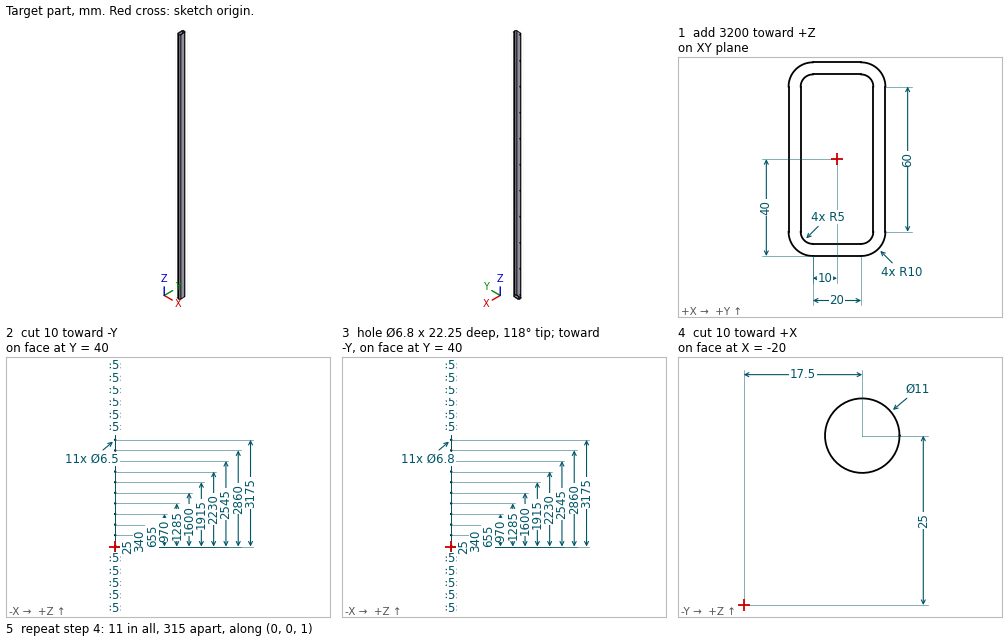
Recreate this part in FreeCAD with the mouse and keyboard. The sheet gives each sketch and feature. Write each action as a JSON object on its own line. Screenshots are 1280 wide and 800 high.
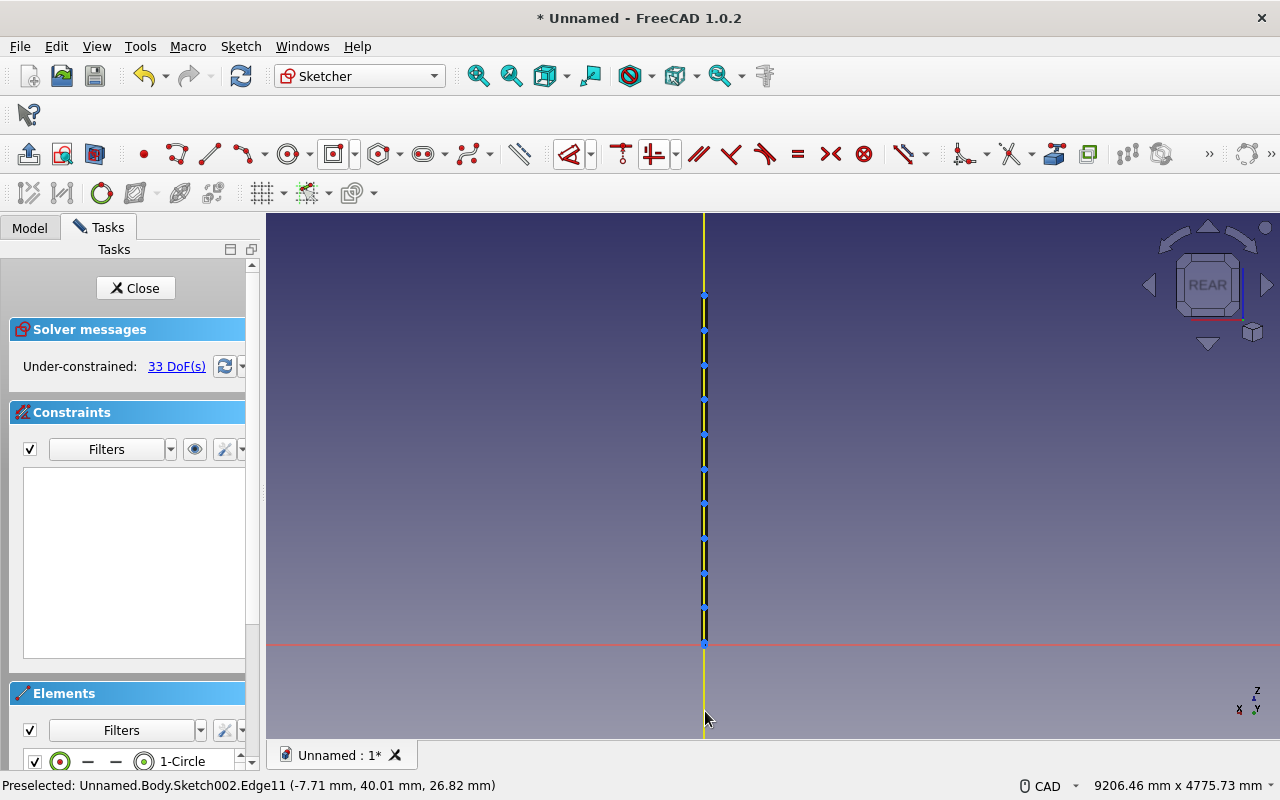
{"action": "scroll", "coordinate": [705, 295], "scroll_direction": "up", "scroll_amount": 14}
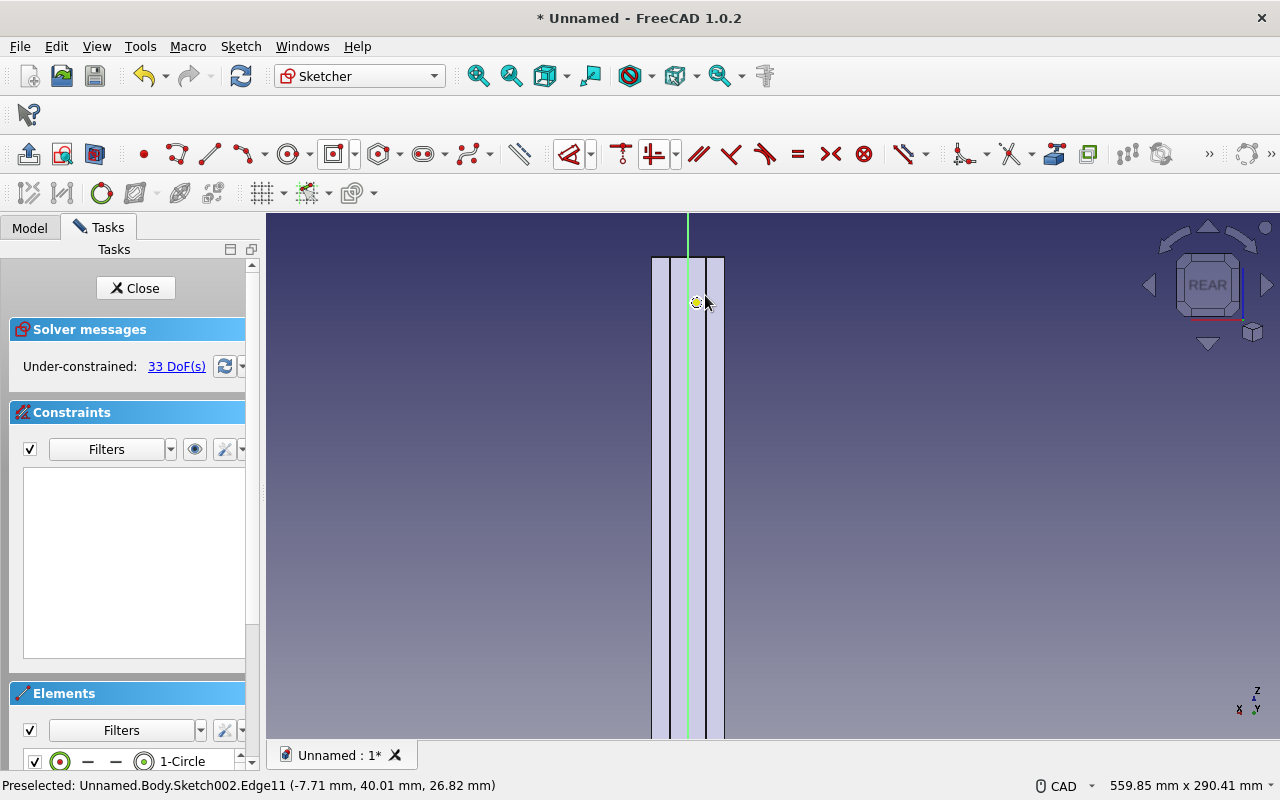
{"action": "left_click", "coordinate": [701, 298]}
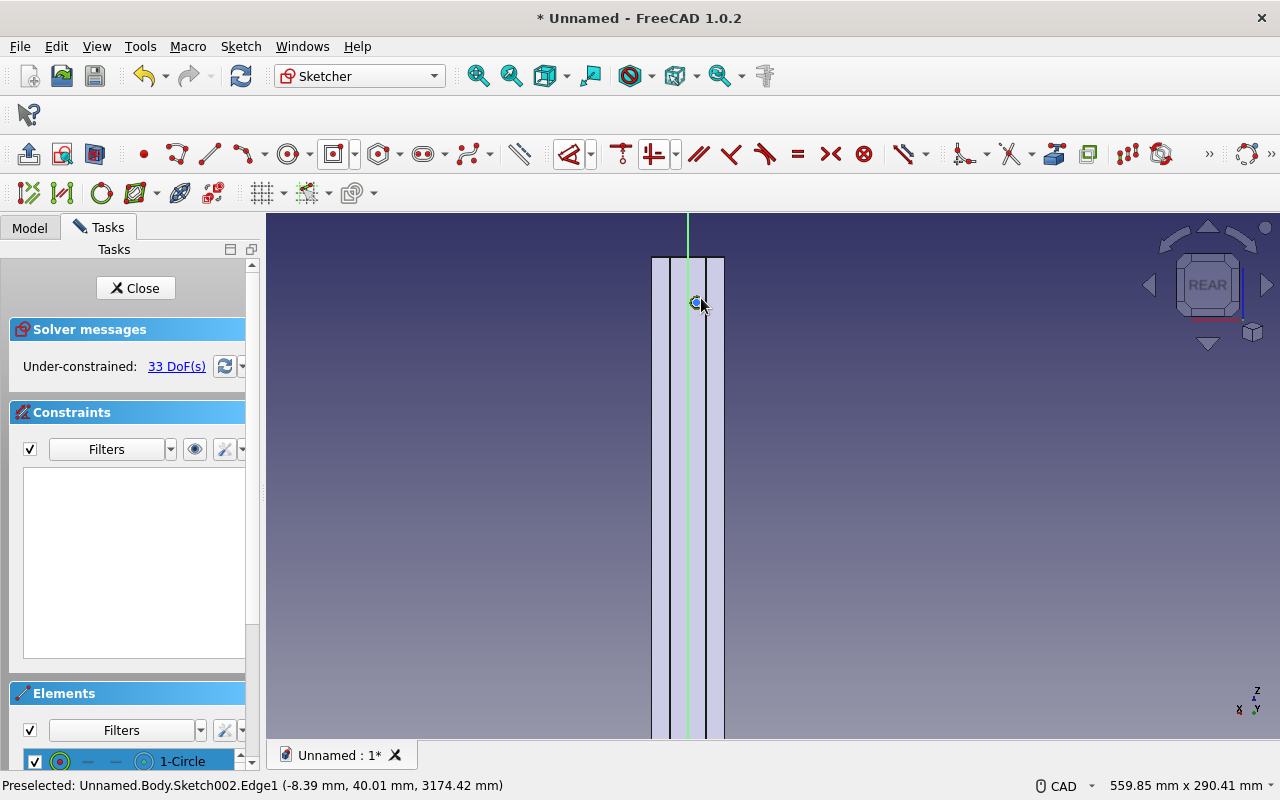
{"action": "scroll", "coordinate": [705, 301], "scroll_direction": "down", "scroll_amount": 14}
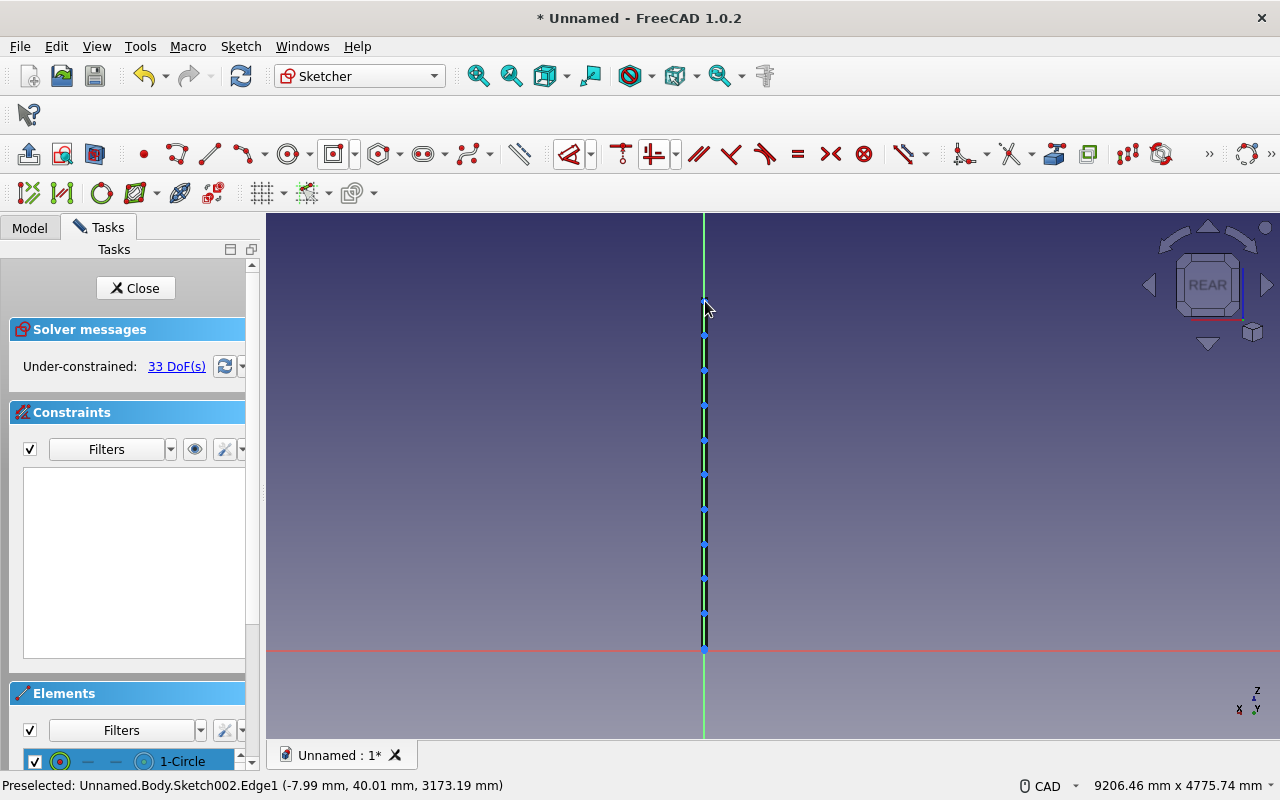
{"action": "scroll", "coordinate": [705, 336], "scroll_direction": "up", "scroll_amount": 14}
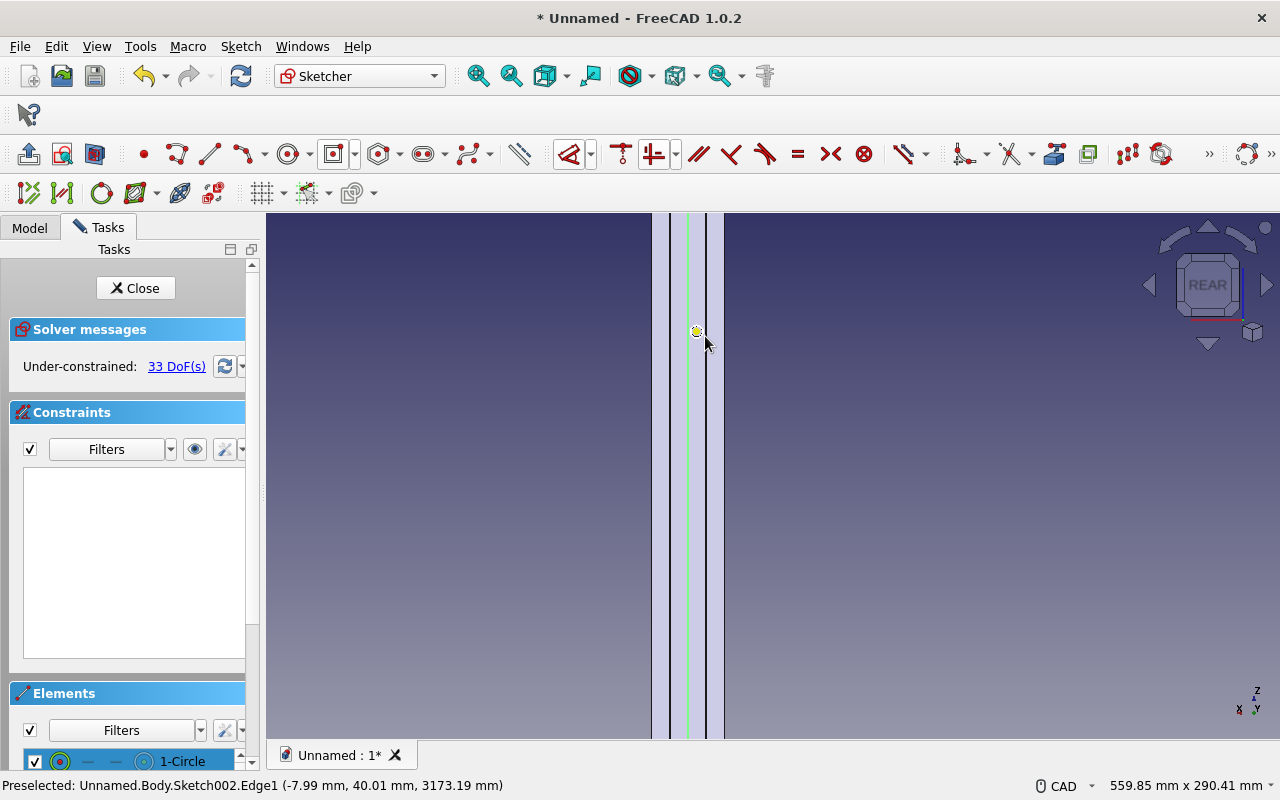
{"action": "left_click", "coordinate": [691, 332]}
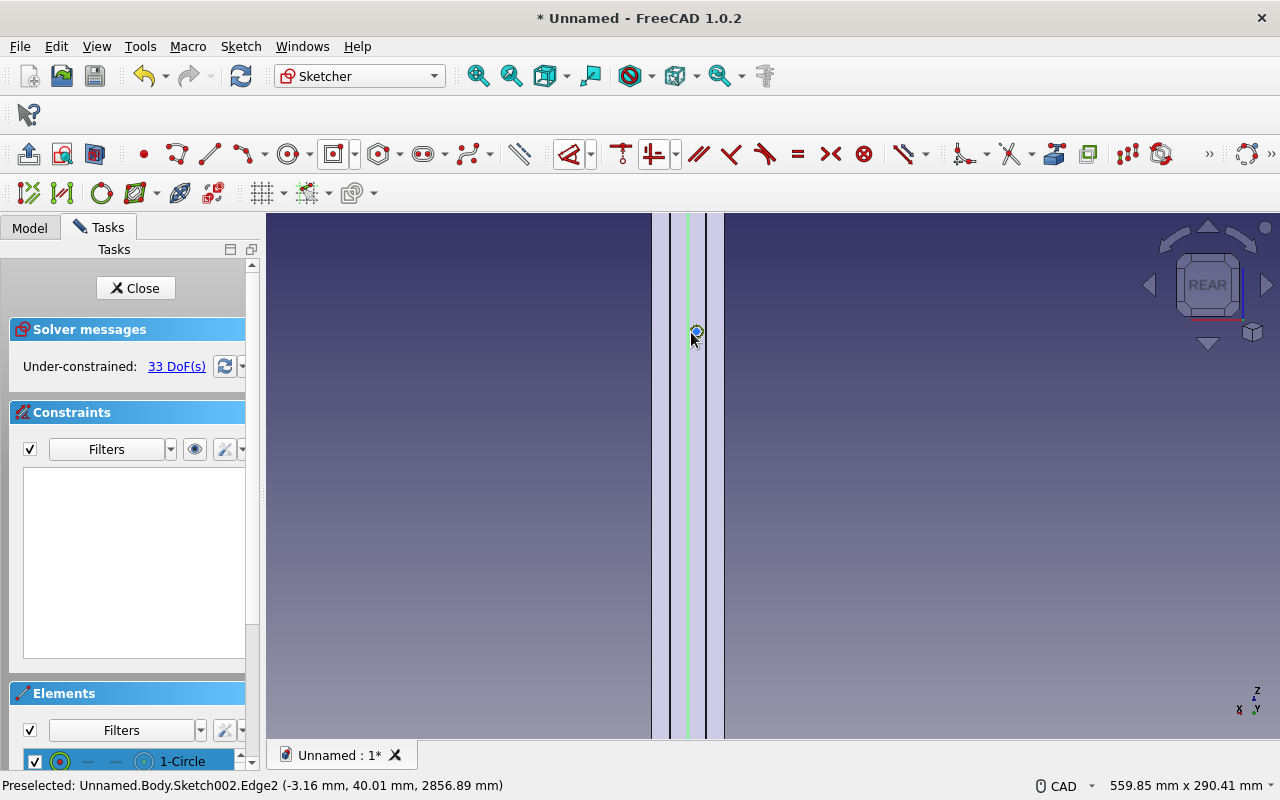
{"action": "scroll", "coordinate": [705, 336], "scroll_direction": "down", "scroll_amount": 14}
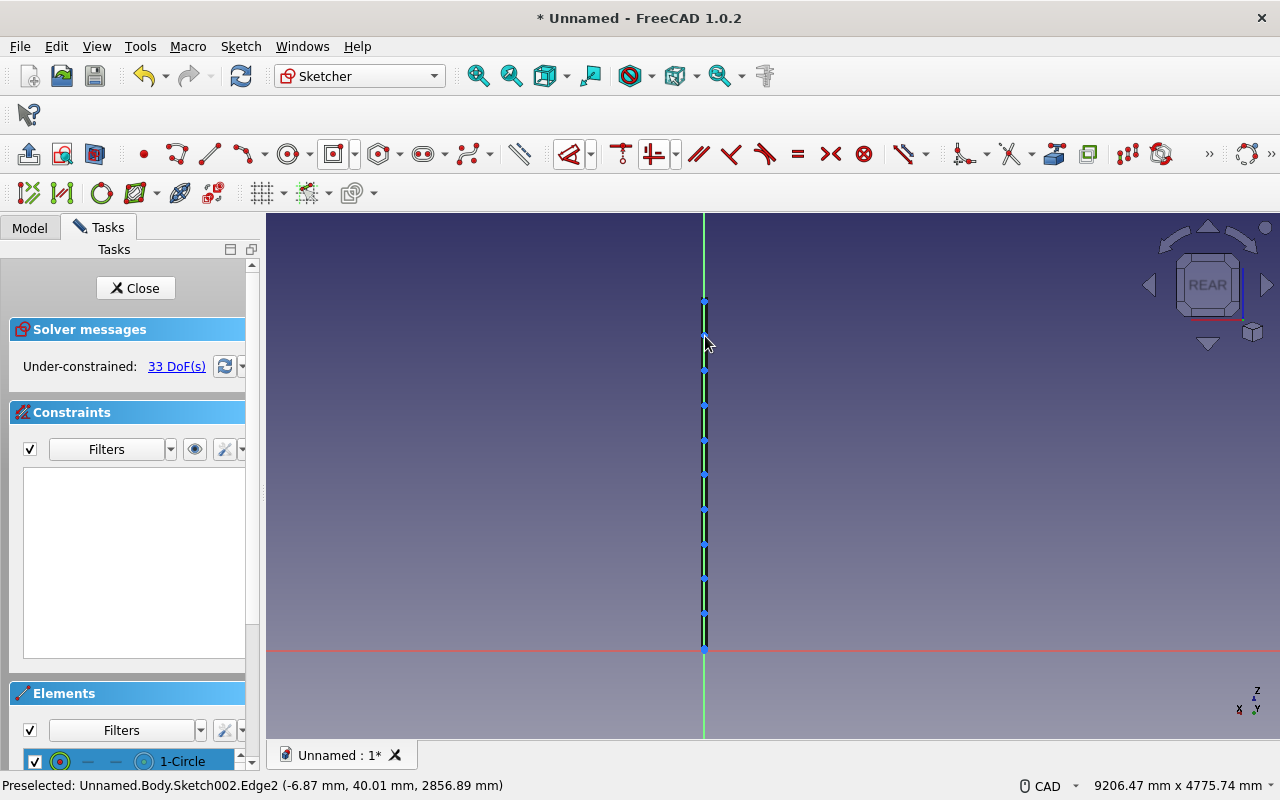
{"action": "scroll", "coordinate": [705, 371], "scroll_direction": "up", "scroll_amount": 14}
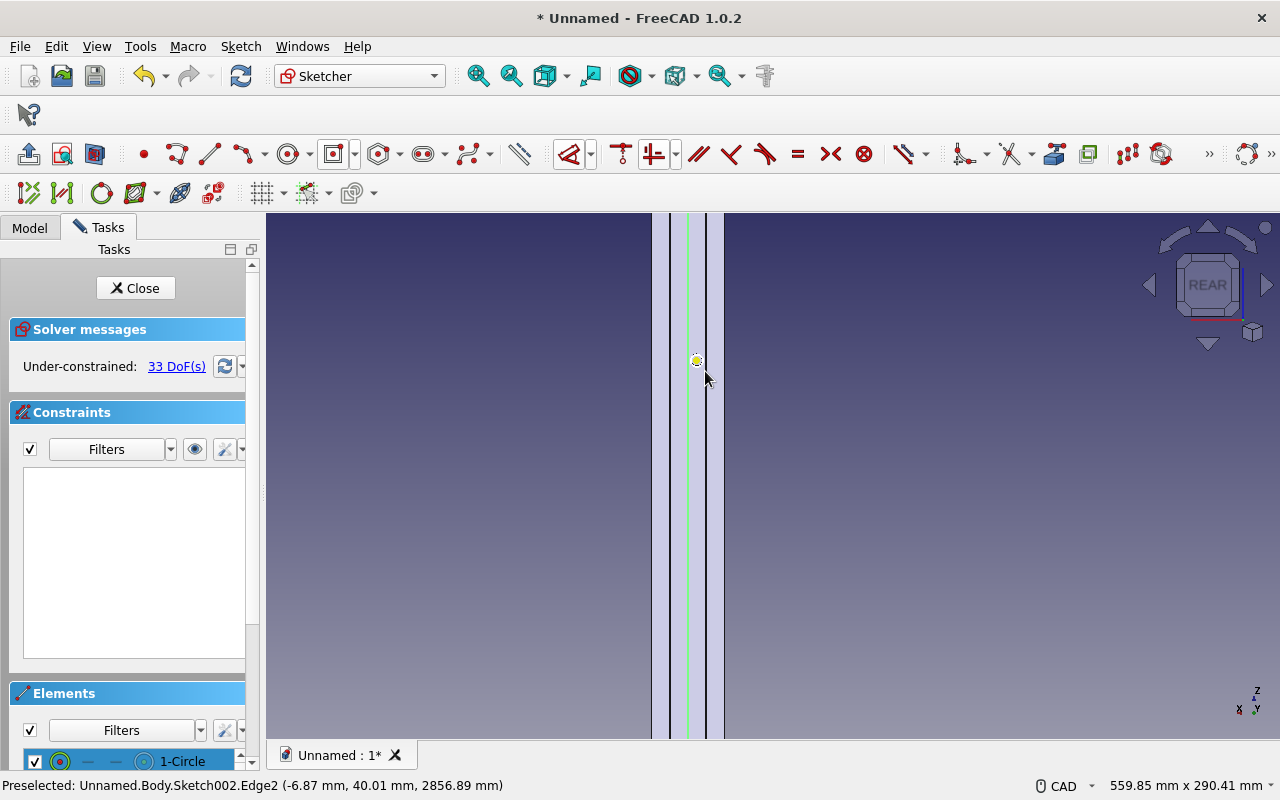
{"action": "left_click", "coordinate": [701, 365]}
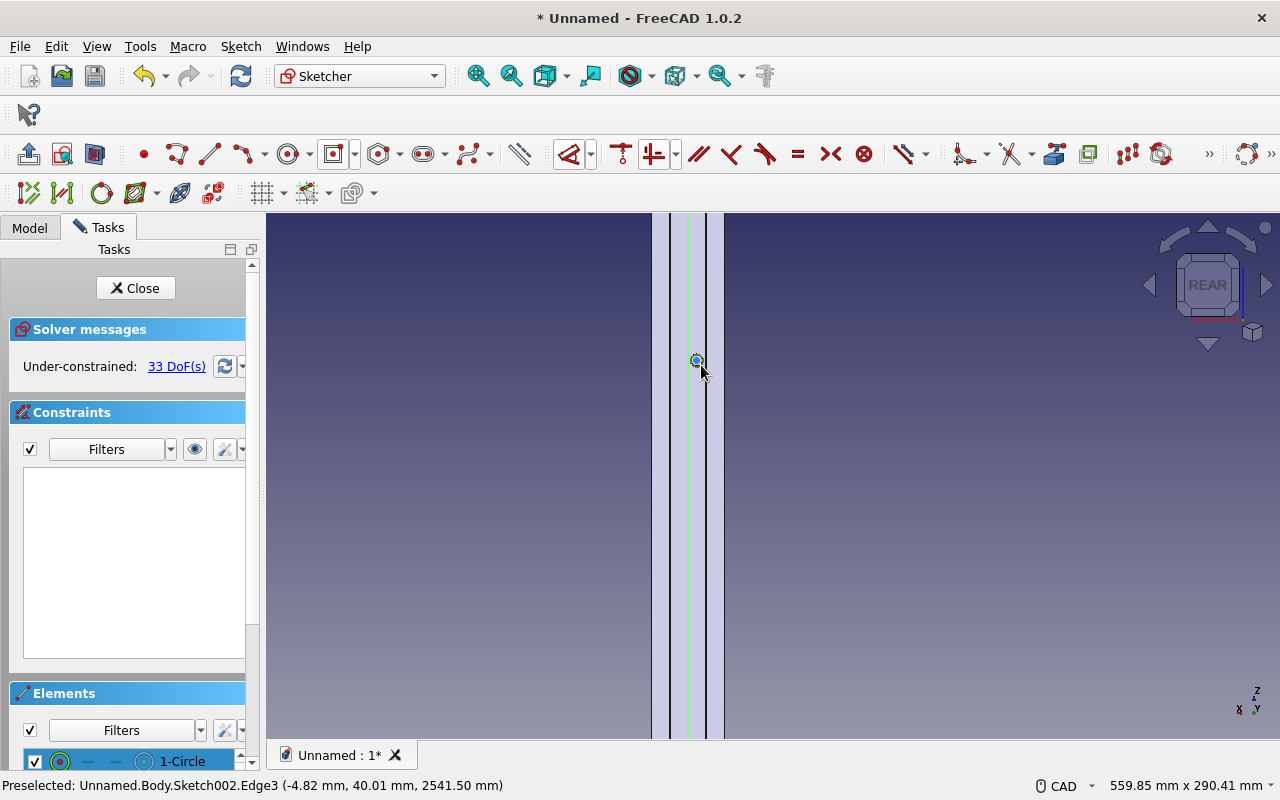
{"action": "scroll", "coordinate": [705, 371], "scroll_direction": "down", "scroll_amount": 14}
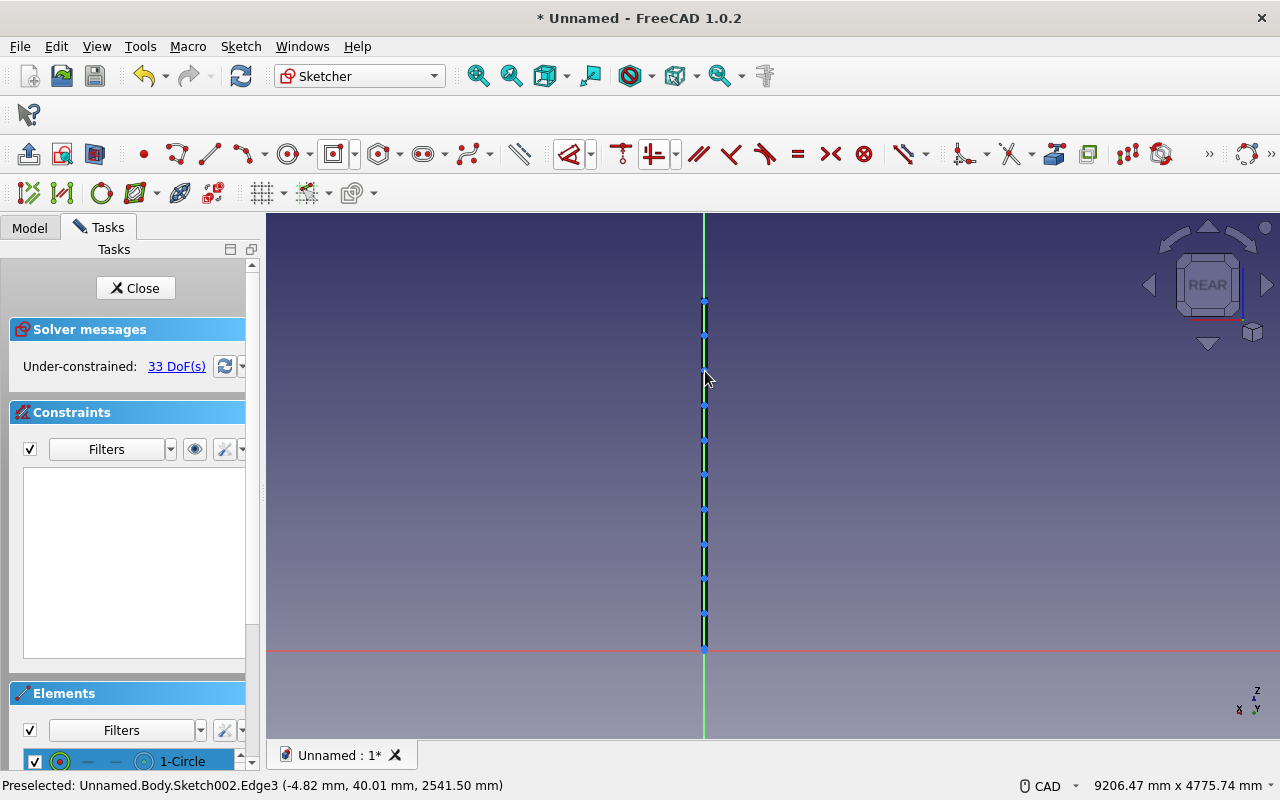
{"action": "scroll", "coordinate": [705, 405], "scroll_direction": "up", "scroll_amount": 14}